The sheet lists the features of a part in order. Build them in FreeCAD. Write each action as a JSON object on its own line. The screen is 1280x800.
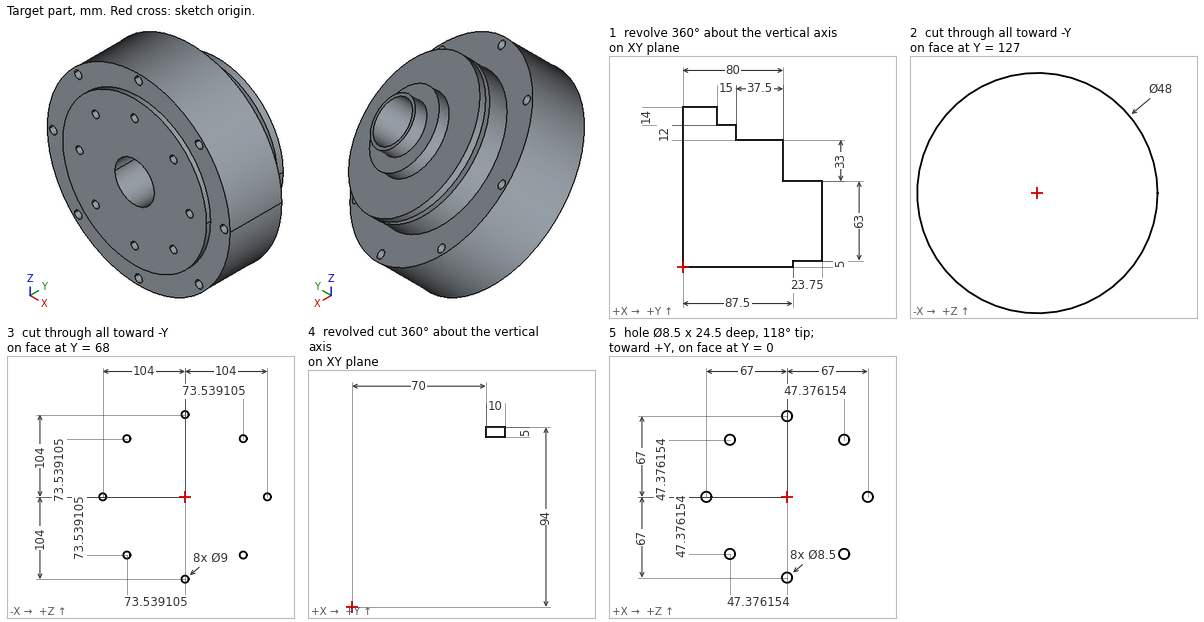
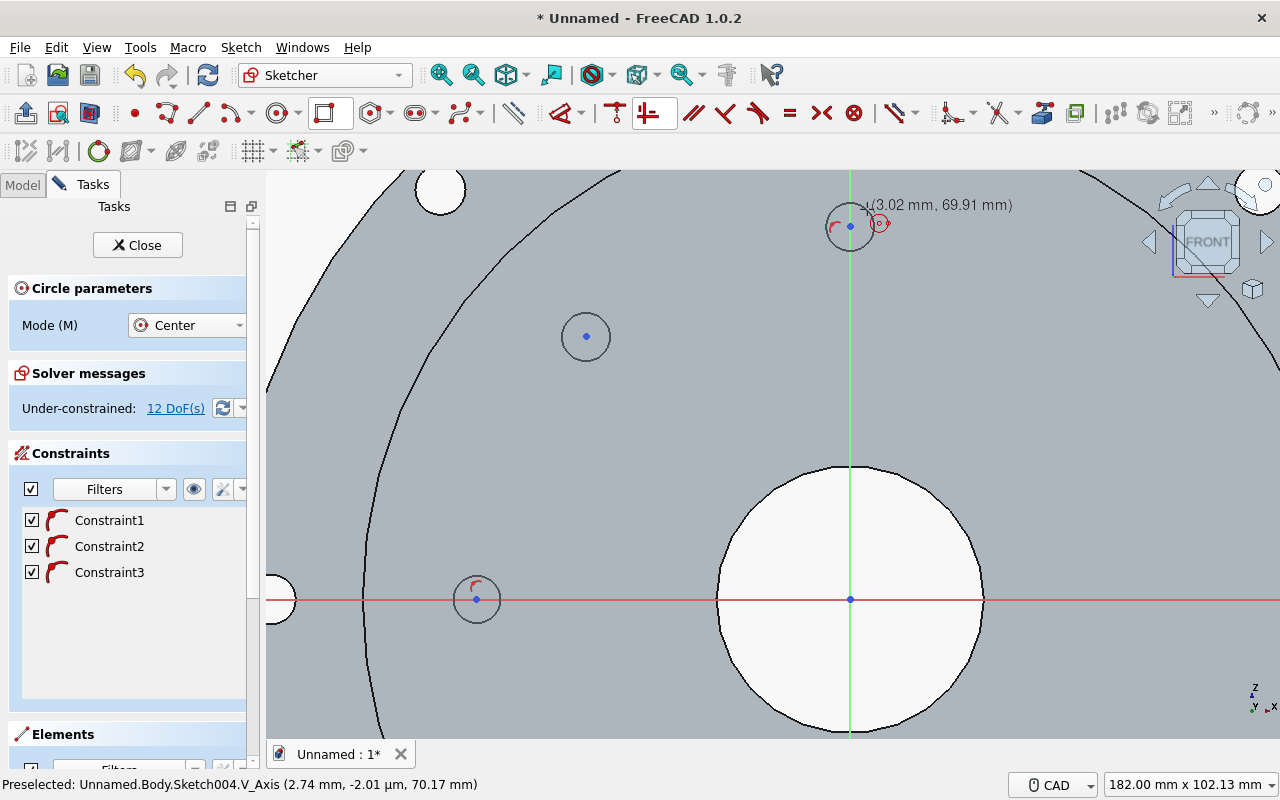
{"action": "left_click", "coordinate": [1114, 336]}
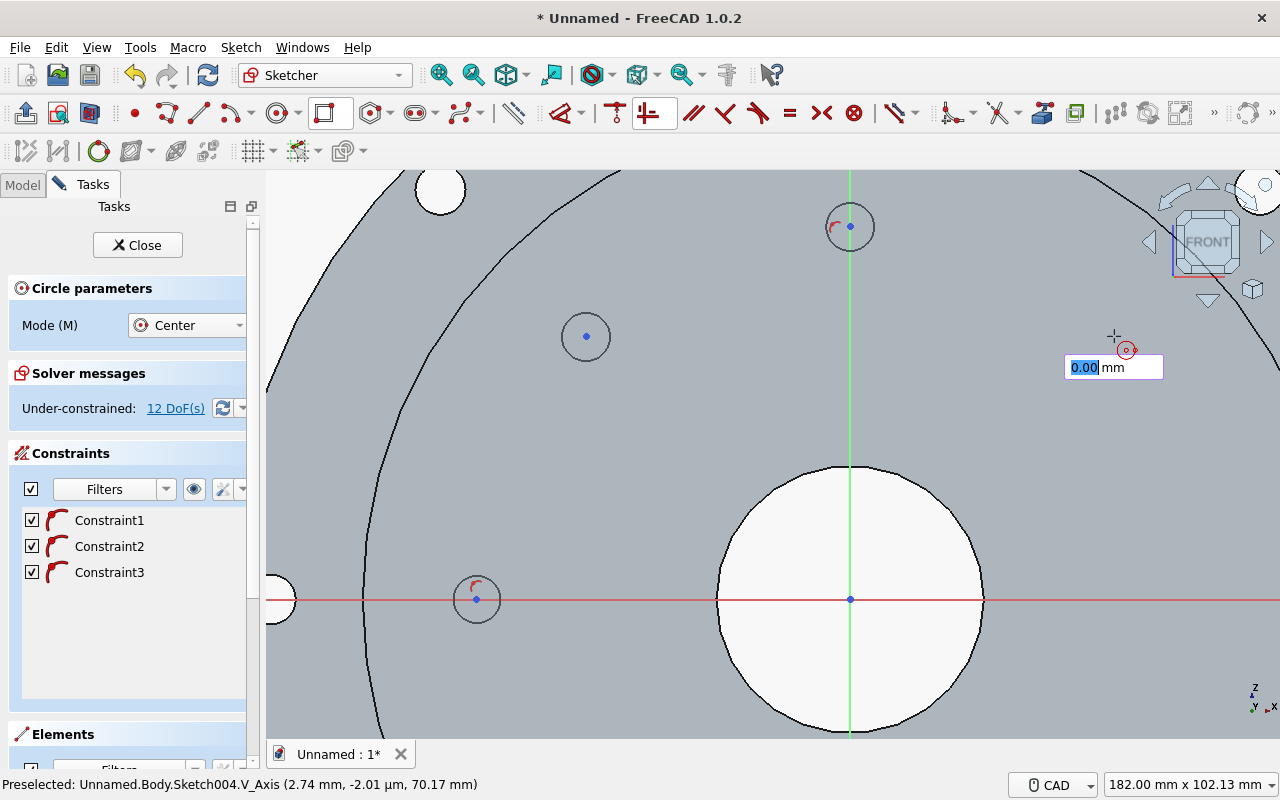
{"action": "scroll", "coordinate": [586, 336], "scroll_direction": "down", "scroll_amount": 4}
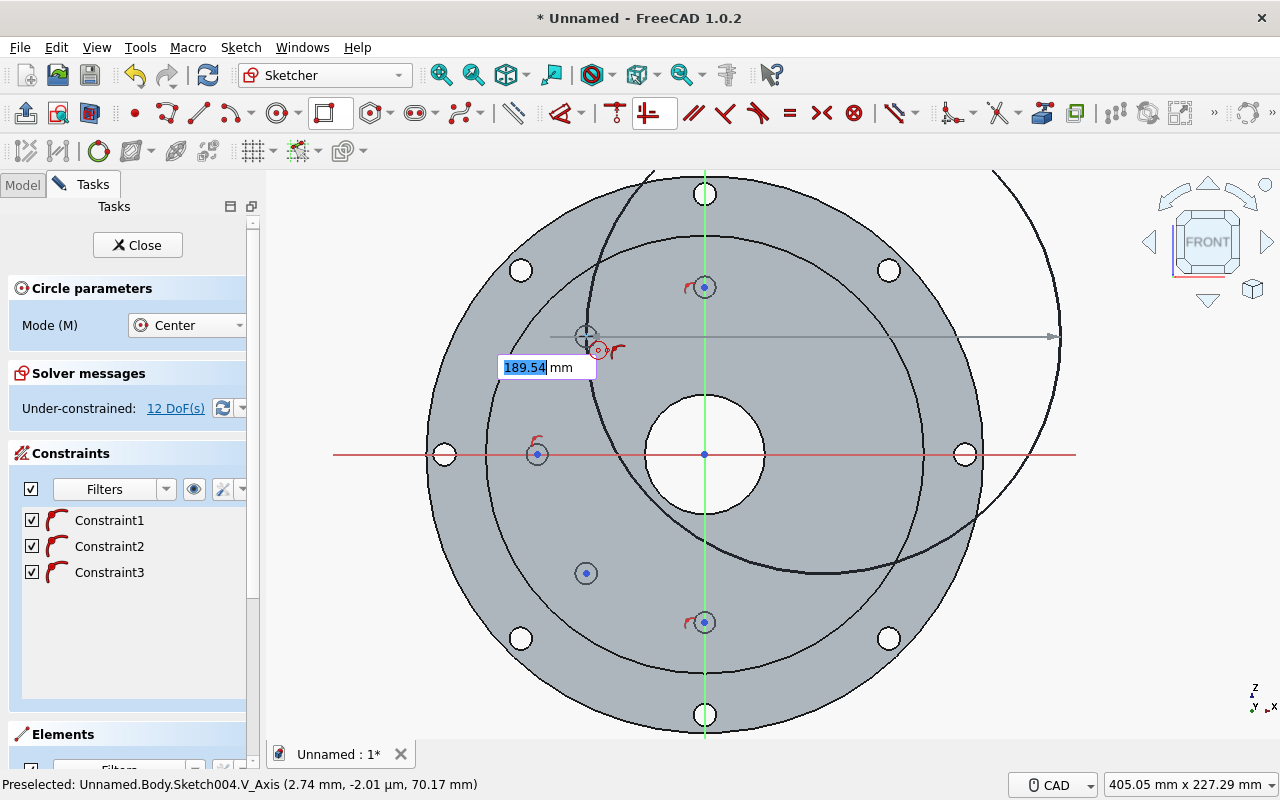
{"action": "scroll", "coordinate": [831, 328], "scroll_direction": "up", "scroll_amount": 3}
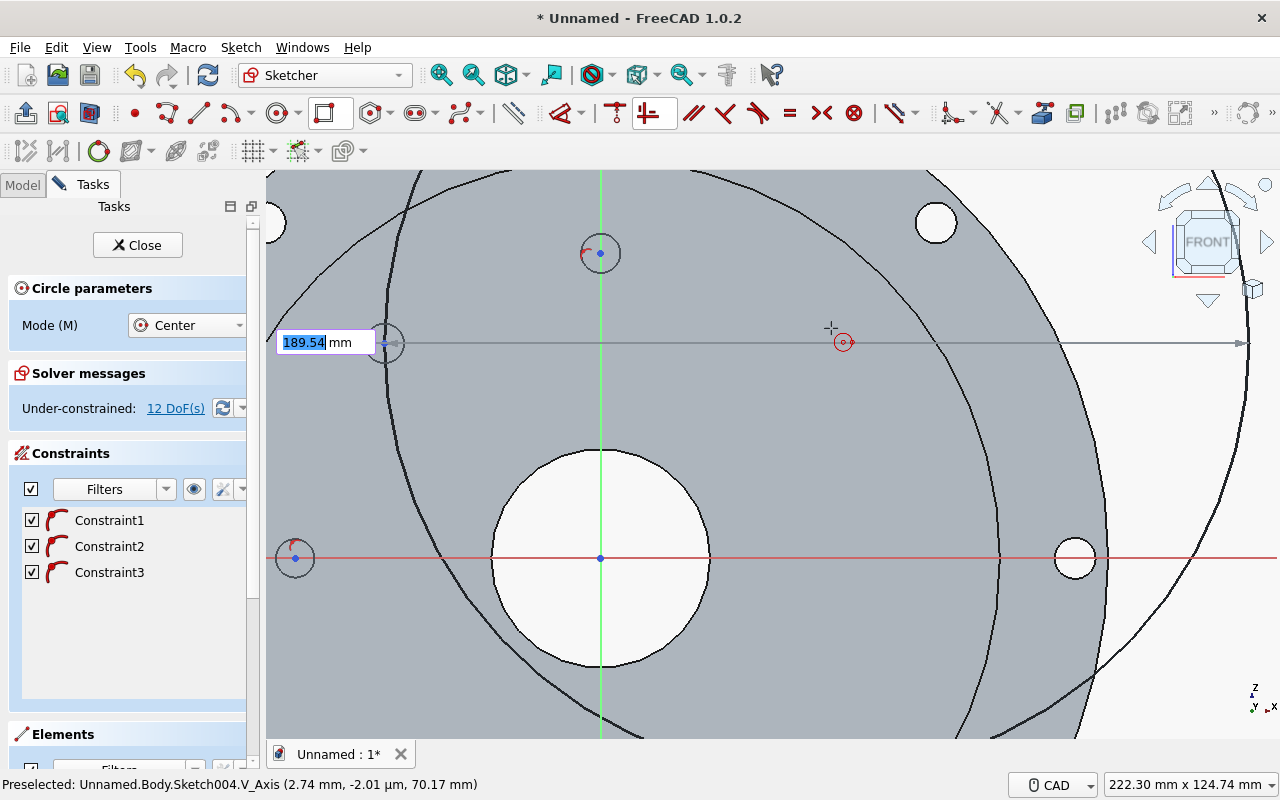
{"action": "left_click", "coordinate": [831, 329]}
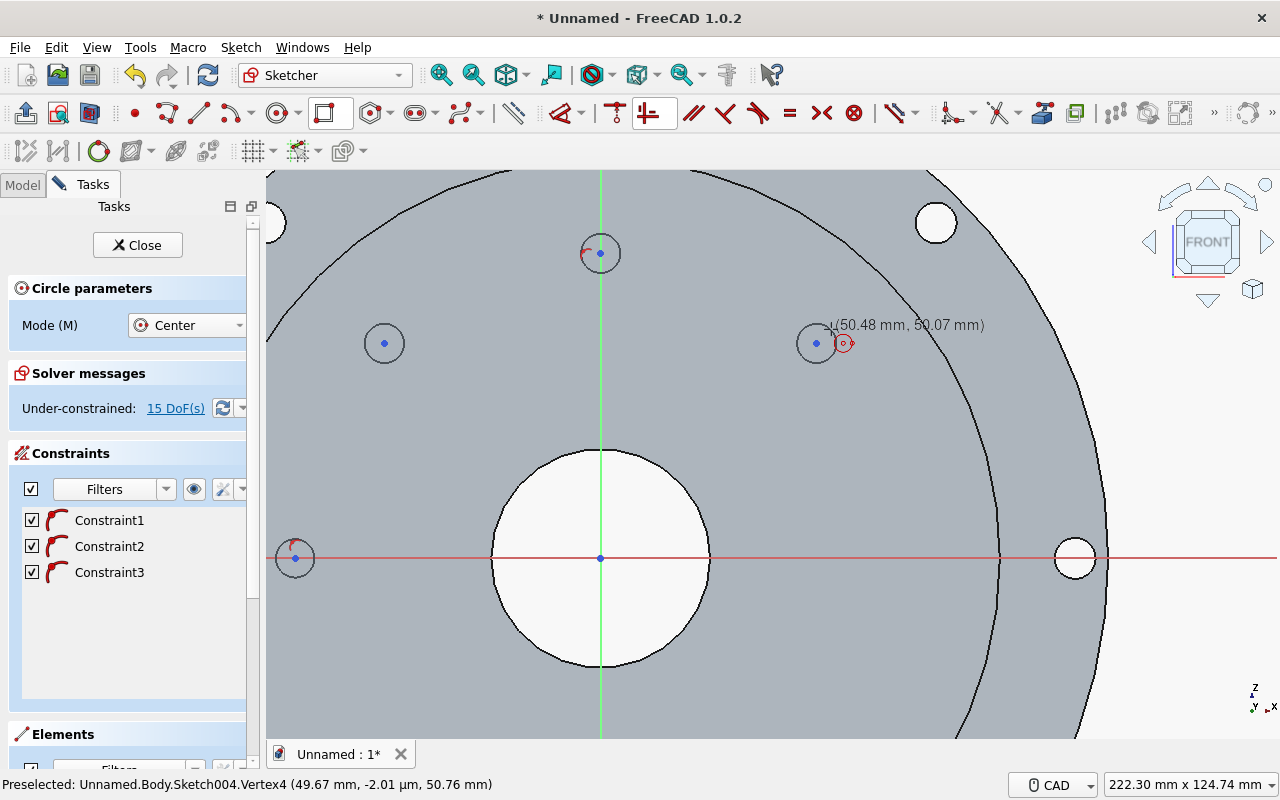
{"action": "left_click", "coordinate": [906, 558]}
{"action": "left_click", "coordinate": [913, 540]}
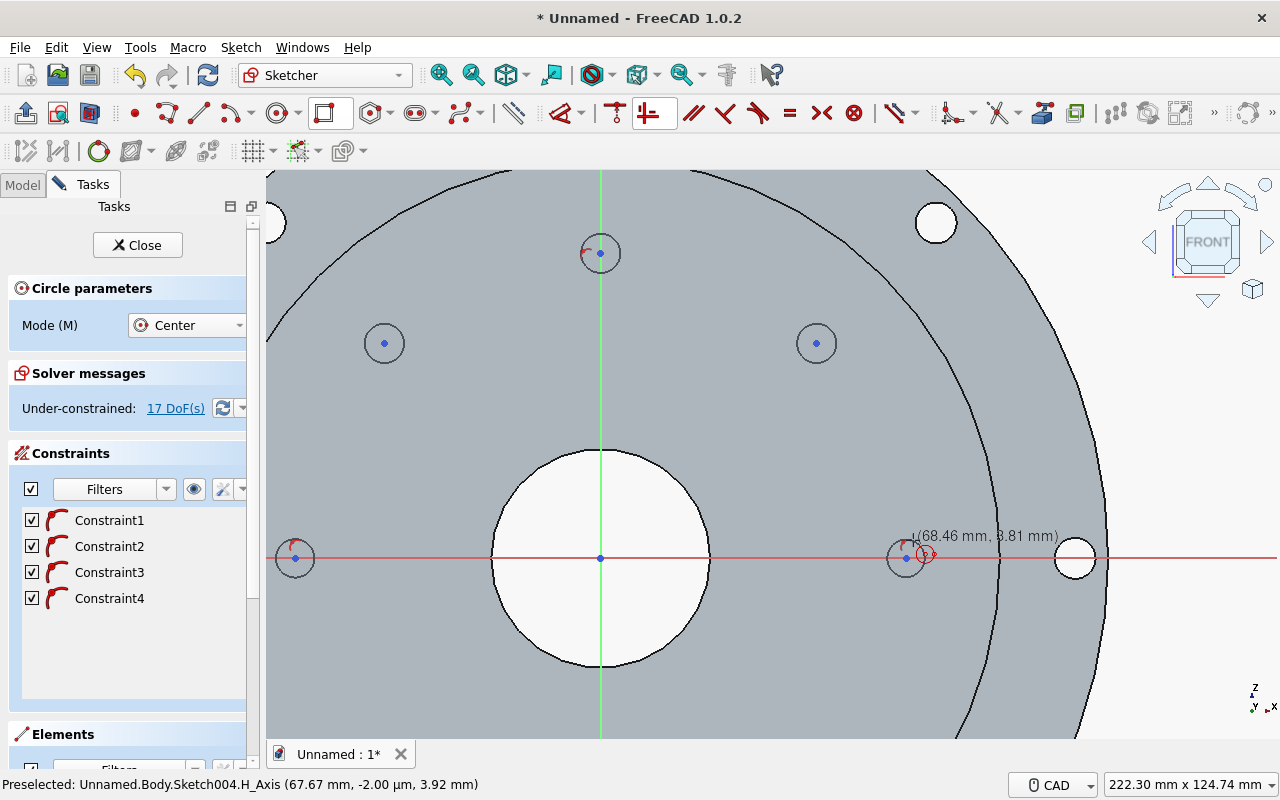
{"action": "scroll", "coordinate": [831, 328], "scroll_direction": "down", "scroll_amount": 3}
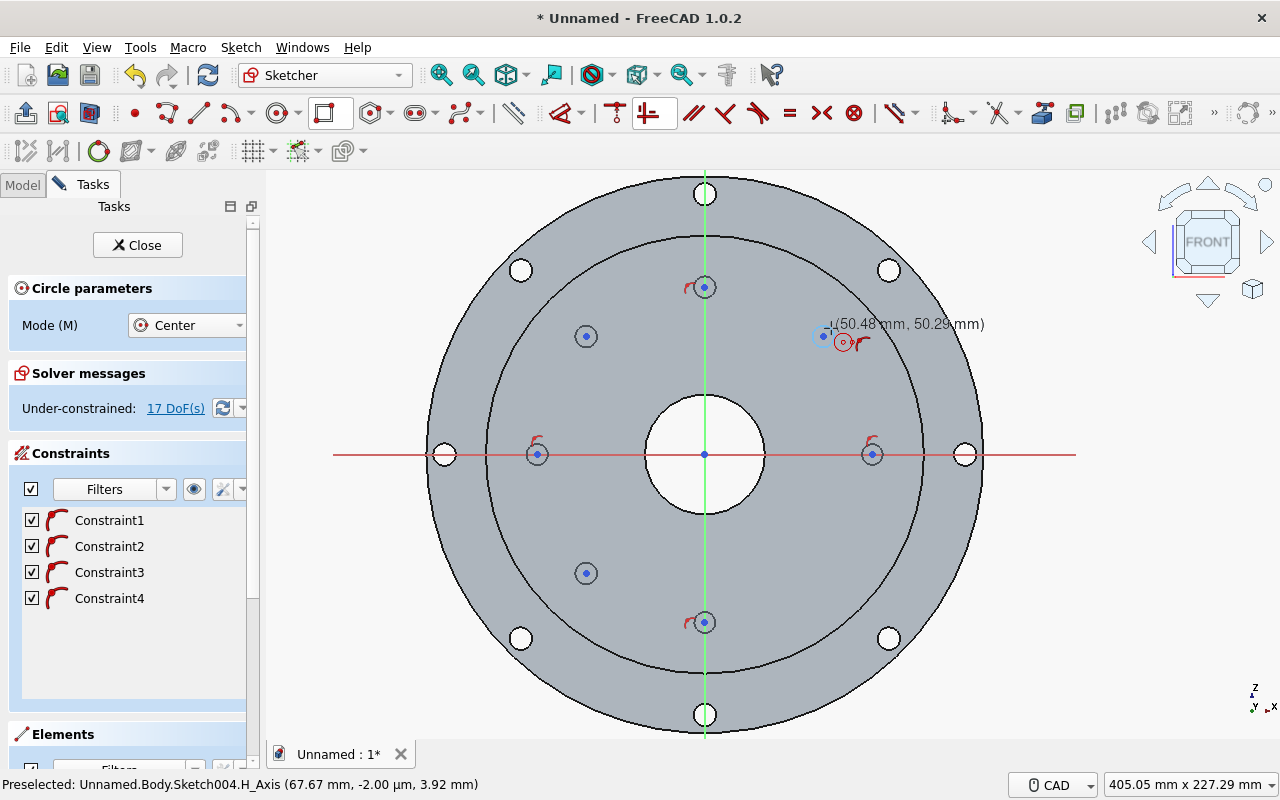
{"action": "scroll", "coordinate": [823, 573], "scroll_direction": "up", "scroll_amount": 4}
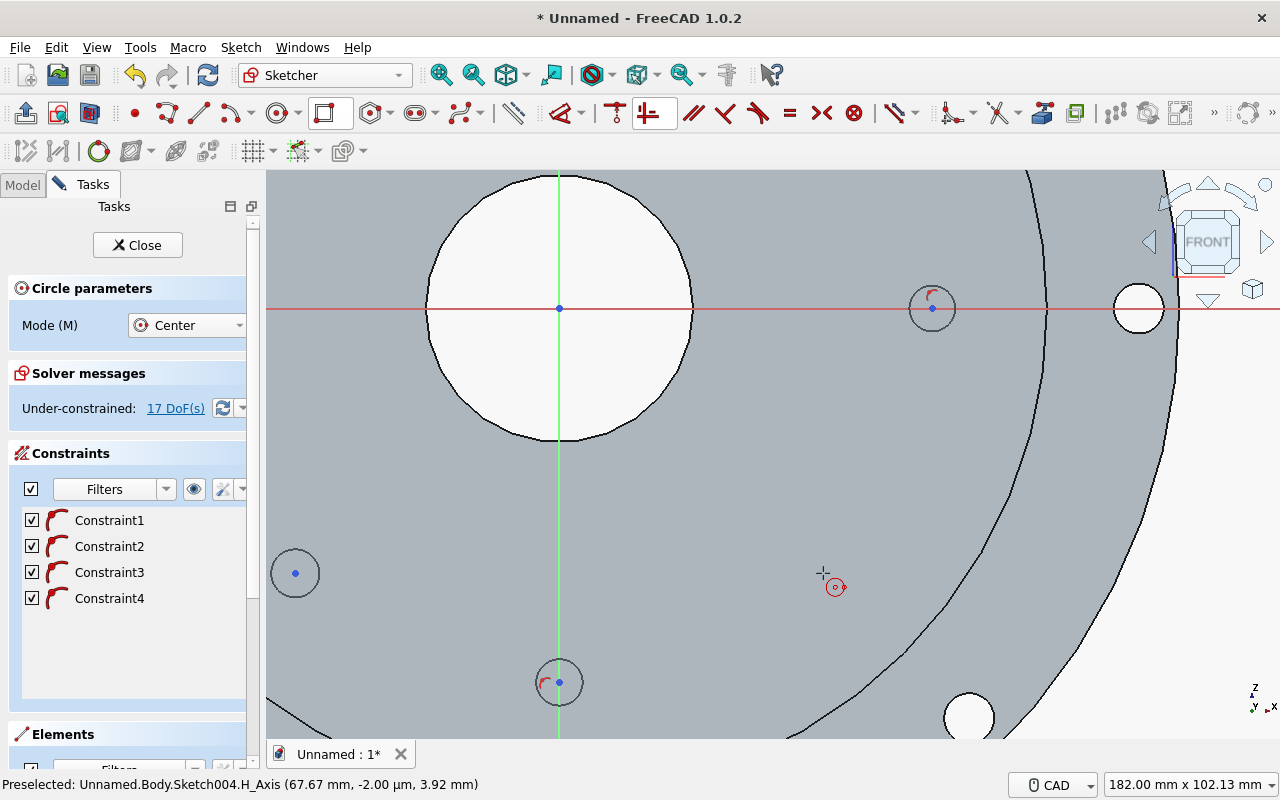
{"action": "left_click", "coordinate": [823, 572]}
{"action": "left_click", "coordinate": [840, 556]}
{"action": "key", "text": "Escape"}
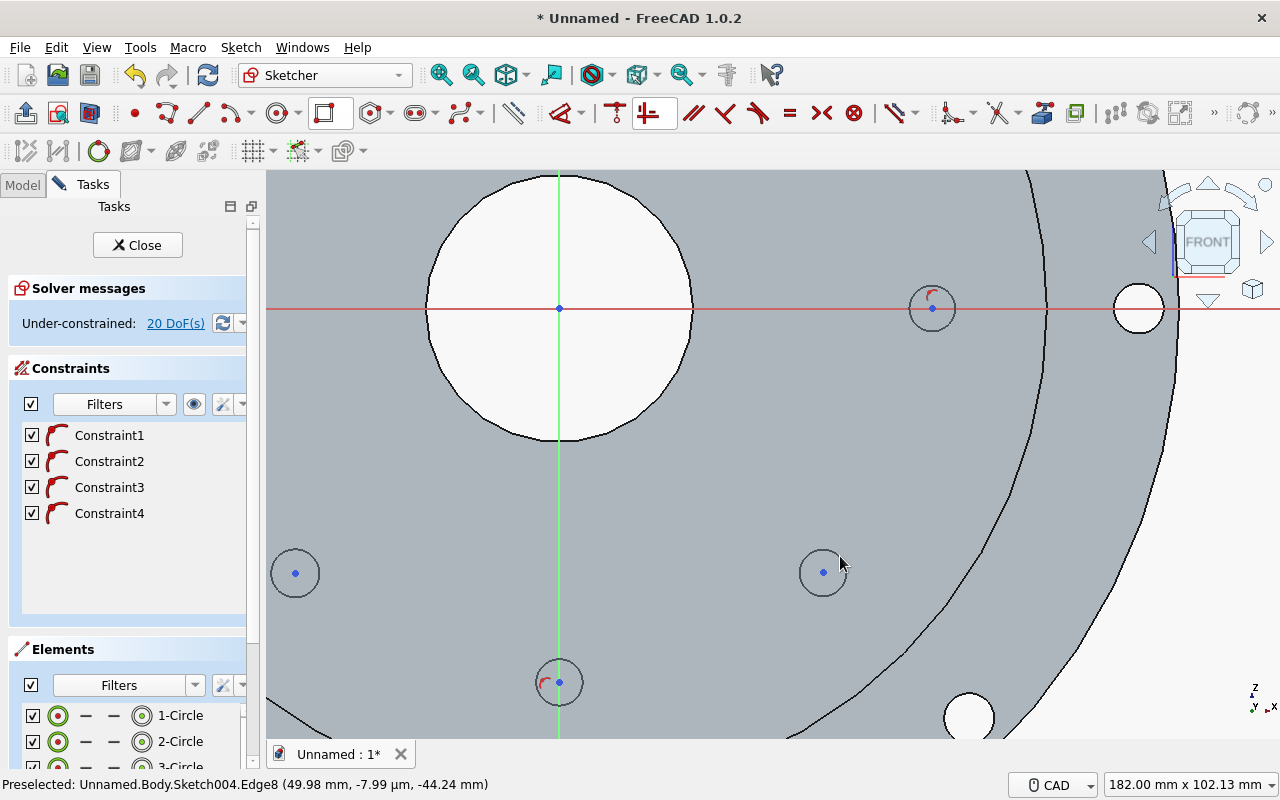
{"action": "left_click", "coordinate": [576, 666]}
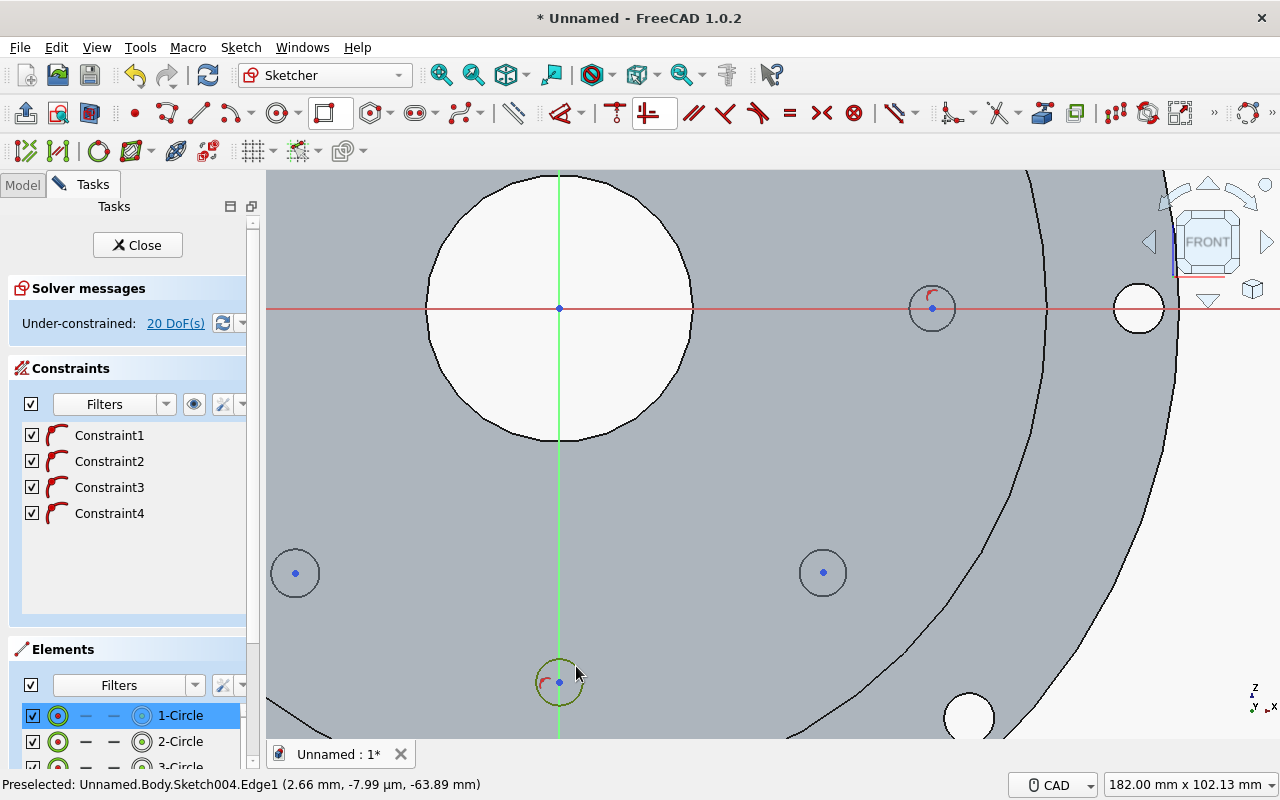
{"action": "left_click", "coordinate": [312, 556]}